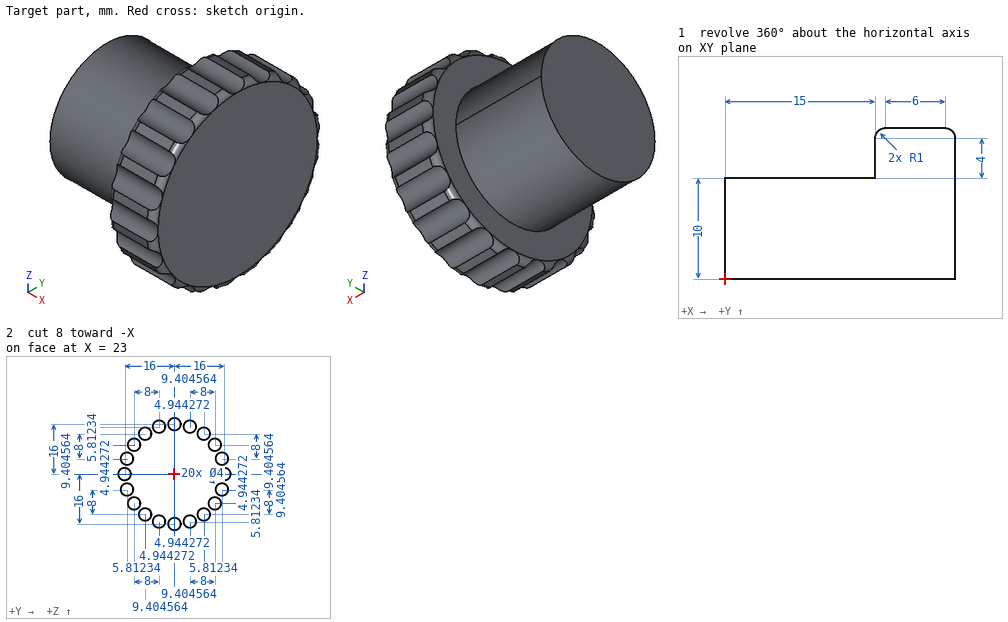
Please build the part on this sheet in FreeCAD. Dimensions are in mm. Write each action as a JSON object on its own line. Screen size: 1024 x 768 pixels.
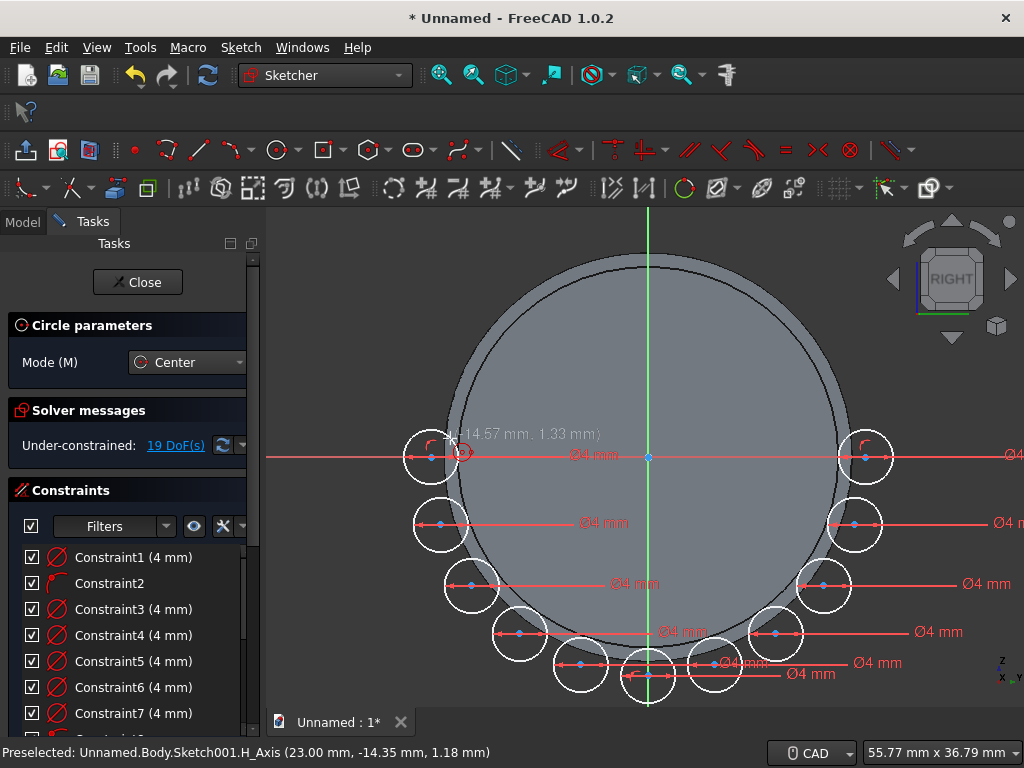
{"action": "left_click", "coordinate": [441, 390]}
{"action": "mouse_move", "coordinate": [460, 371]}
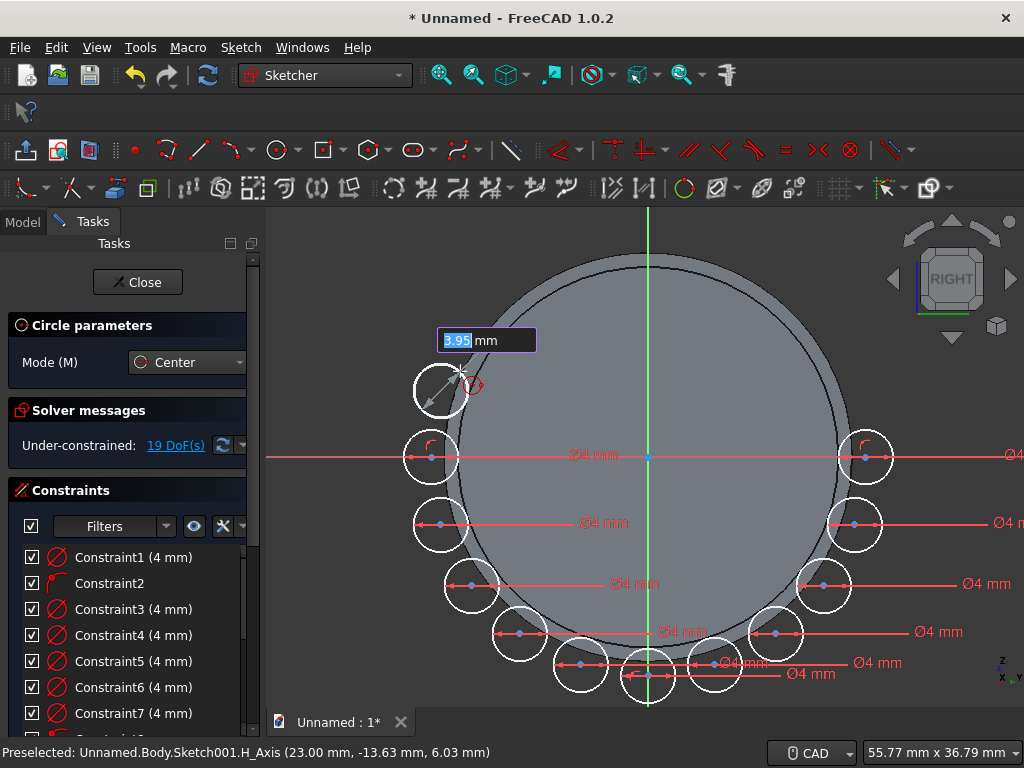
{"action": "type", "text": "4"}
{"action": "key", "text": "Return"}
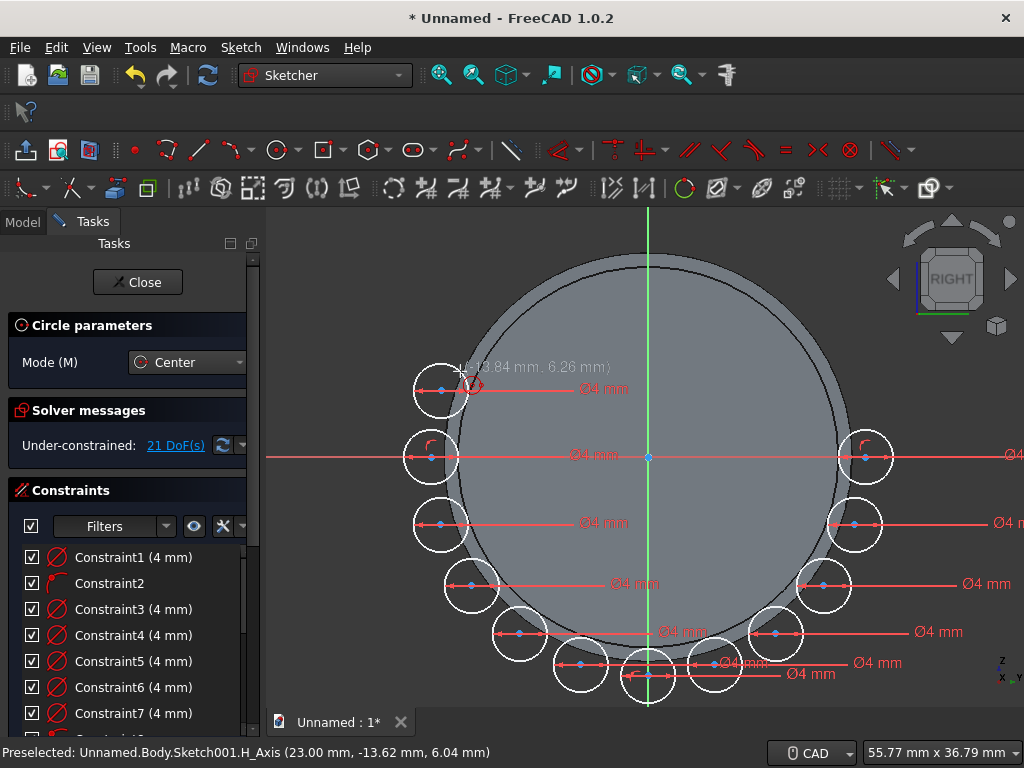
{"action": "left_click", "coordinate": [472, 329]}
{"action": "mouse_move", "coordinate": [491, 310]}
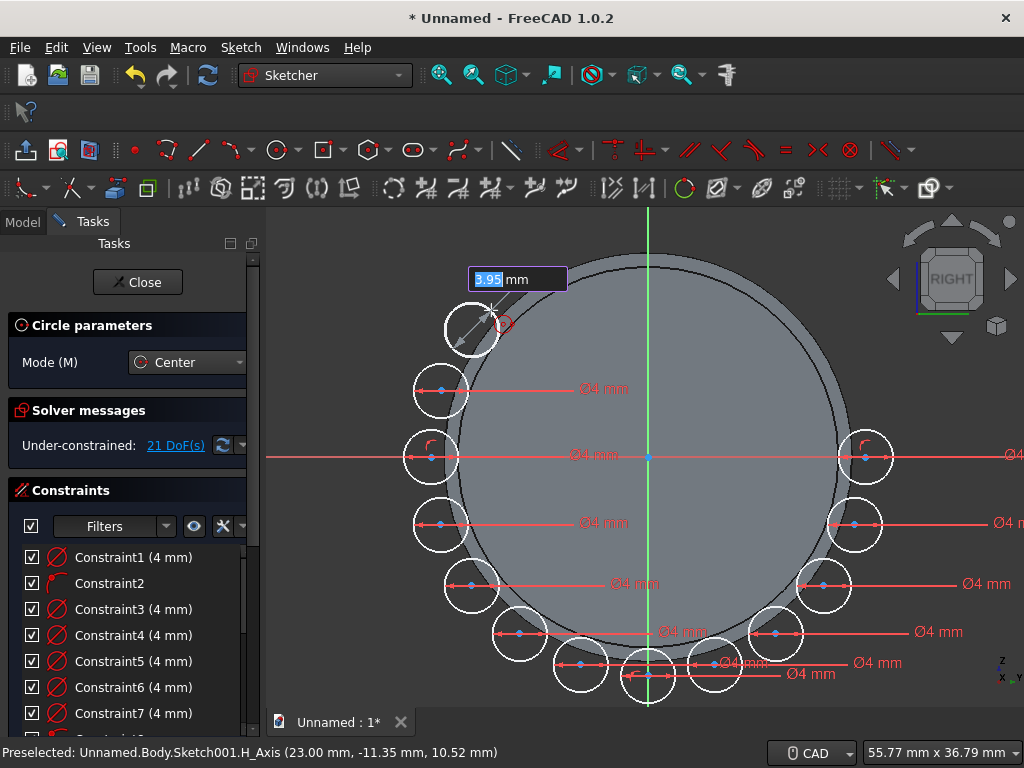
{"action": "type", "text": "4"}
{"action": "key", "text": "Return"}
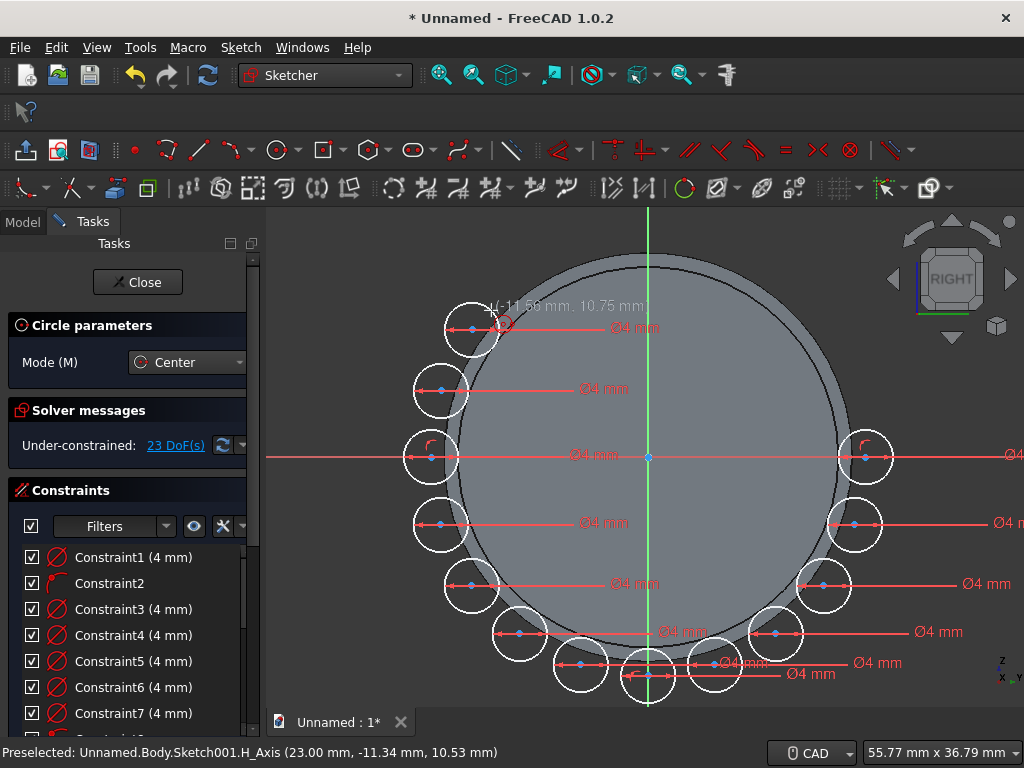
{"action": "left_click", "coordinate": [520, 281]}
{"action": "mouse_move", "coordinate": [539, 262]}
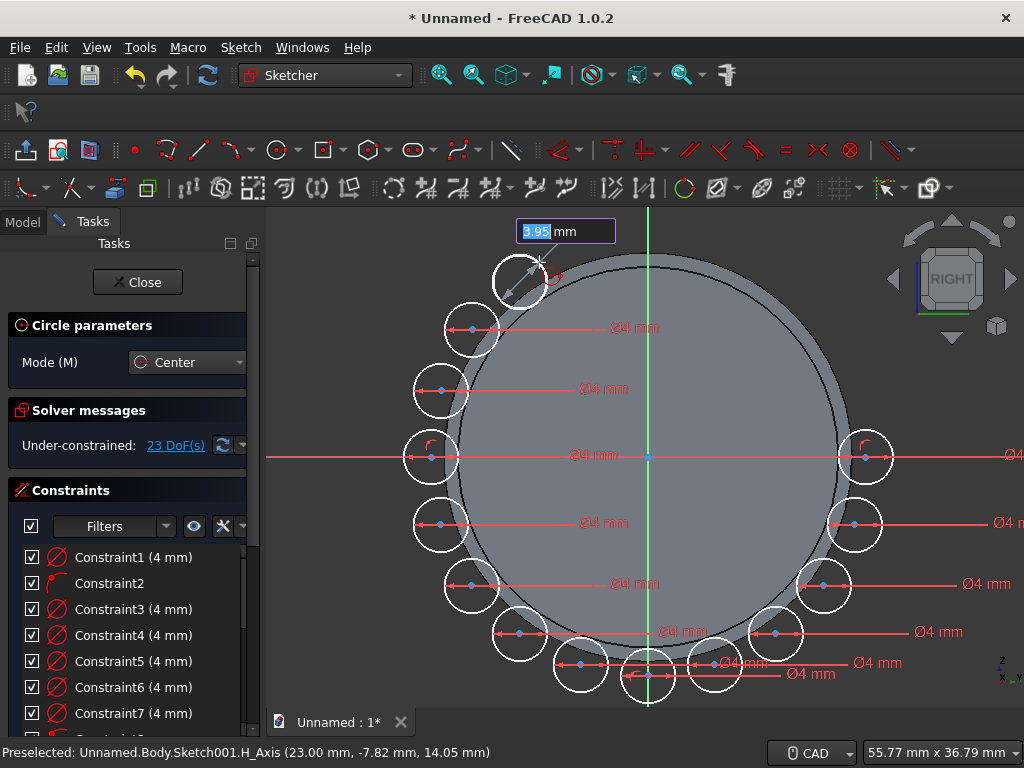
{"action": "type", "text": "4"}
{"action": "key", "text": "Return"}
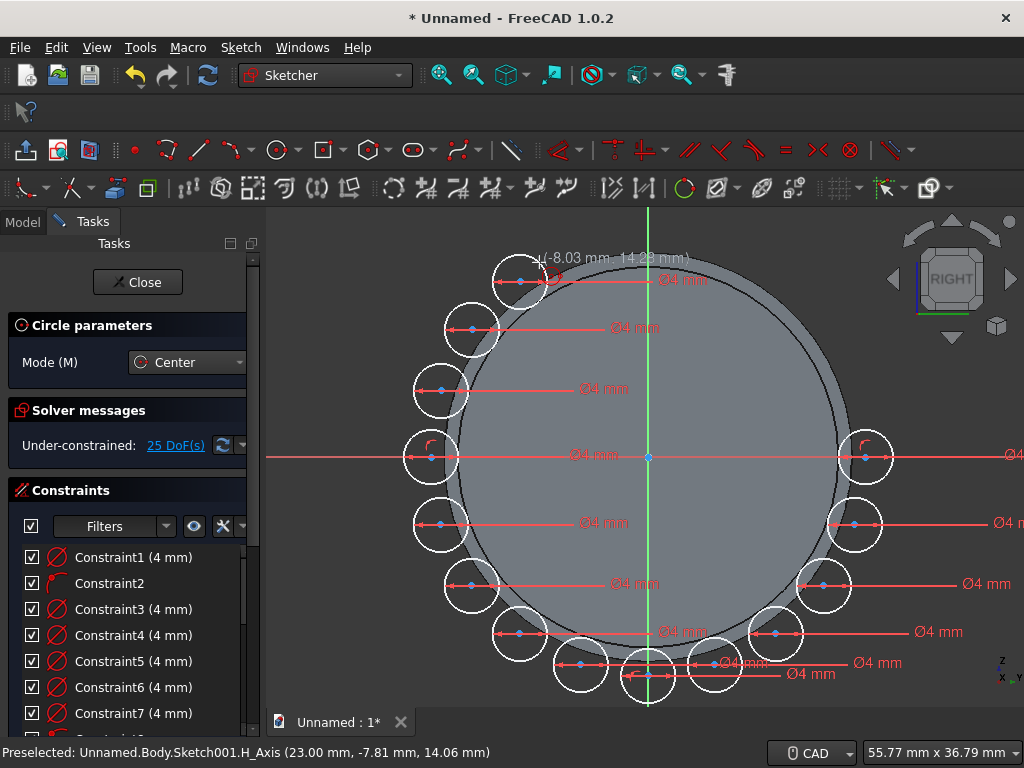
{"action": "left_click", "coordinate": [581, 250]}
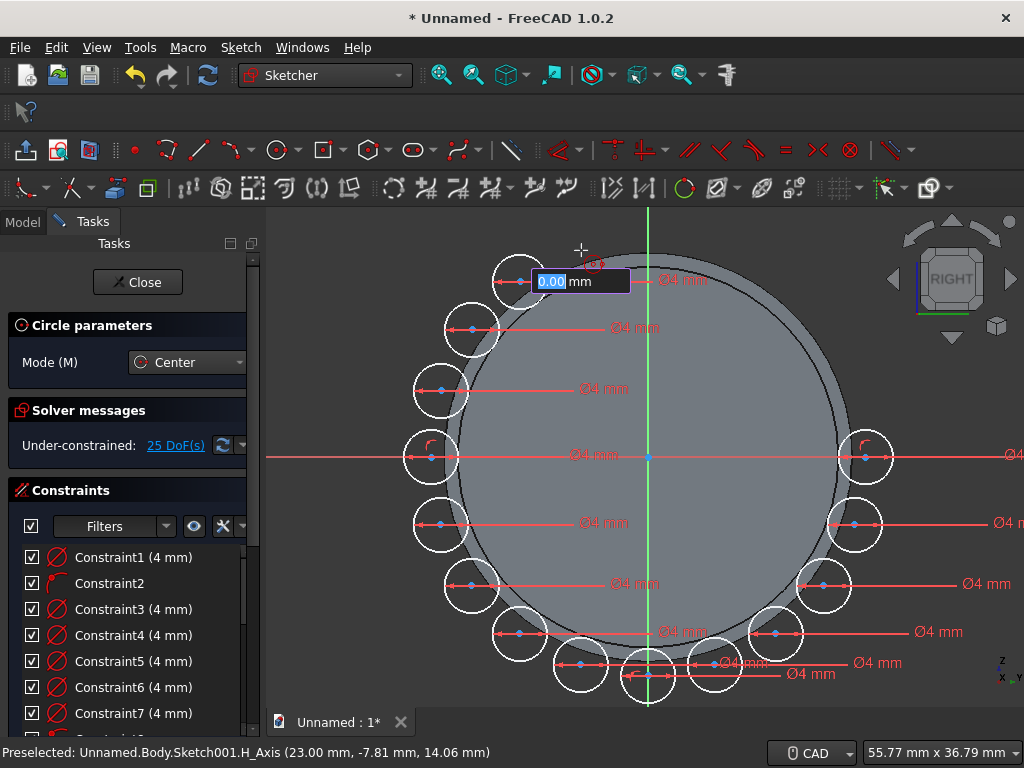
{"action": "scroll", "coordinate": [431, 457], "scroll_direction": "down", "scroll_amount": 2}
{"action": "mouse_move", "coordinate": [544, 306]}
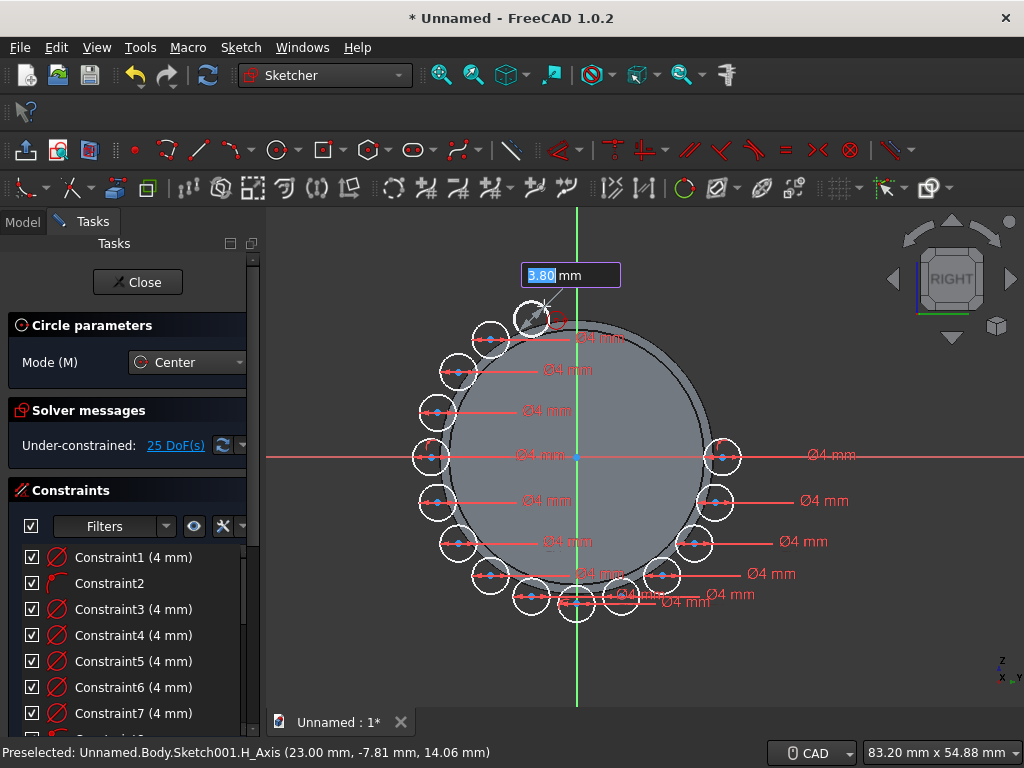
{"action": "type", "text": "4"}
{"action": "key", "text": "Return"}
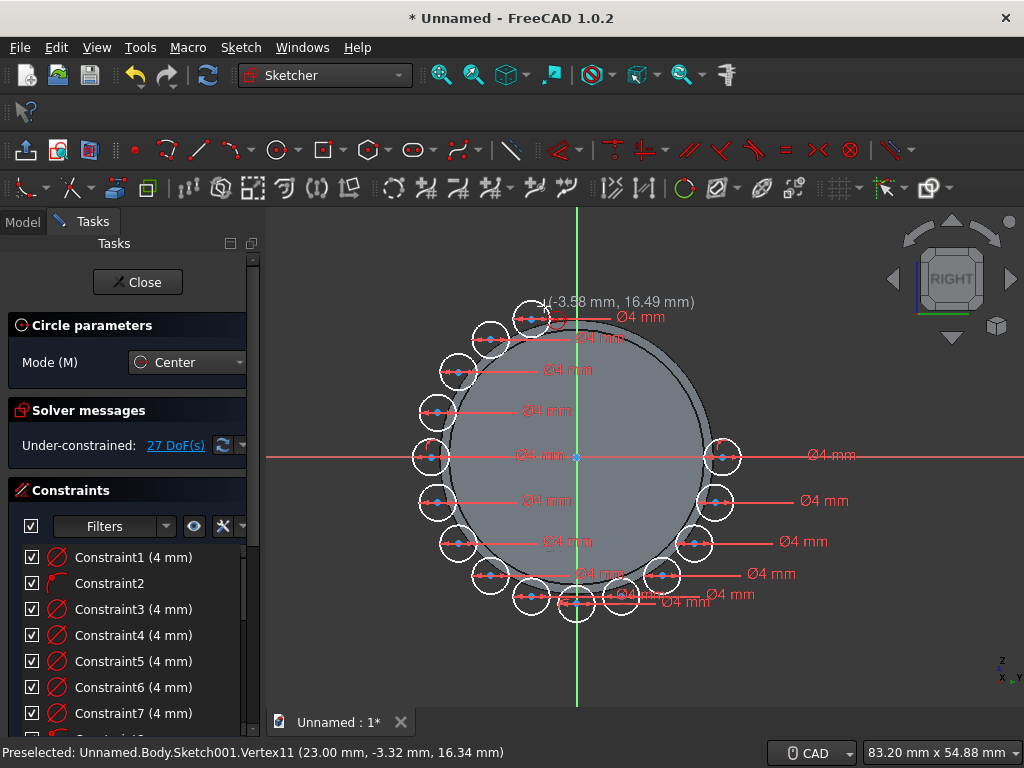
{"action": "scroll", "coordinate": [577, 311], "scroll_direction": "up", "scroll_amount": 2}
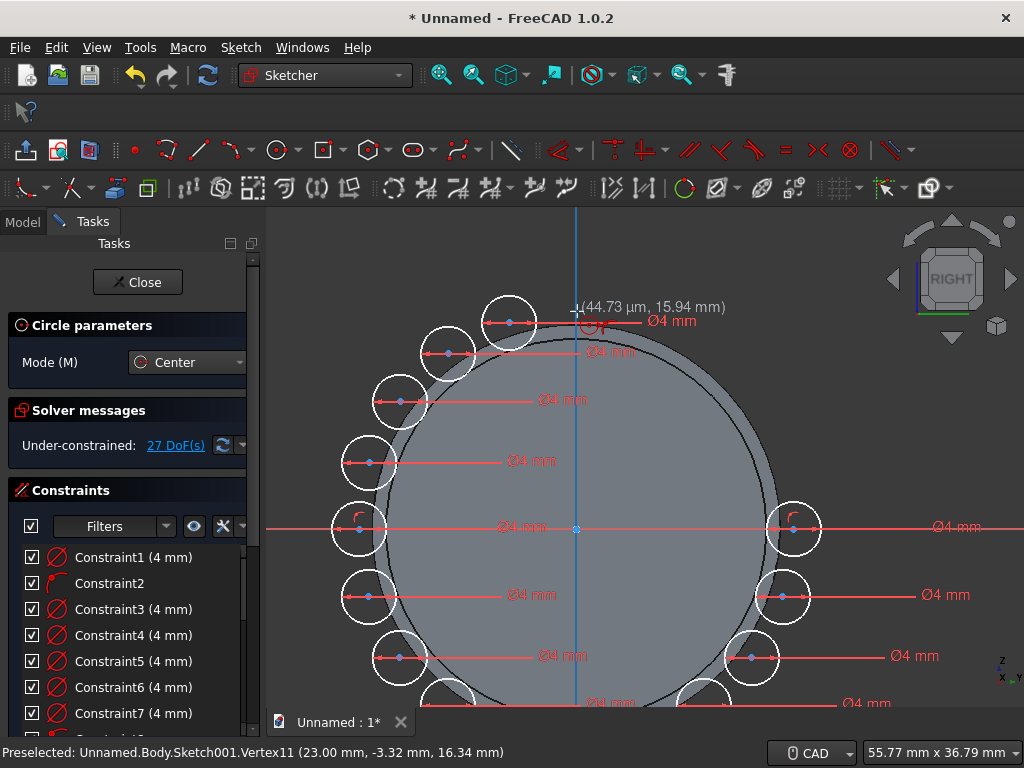
{"action": "left_click", "coordinate": [576, 312]}
{"action": "mouse_move", "coordinate": [595, 292]}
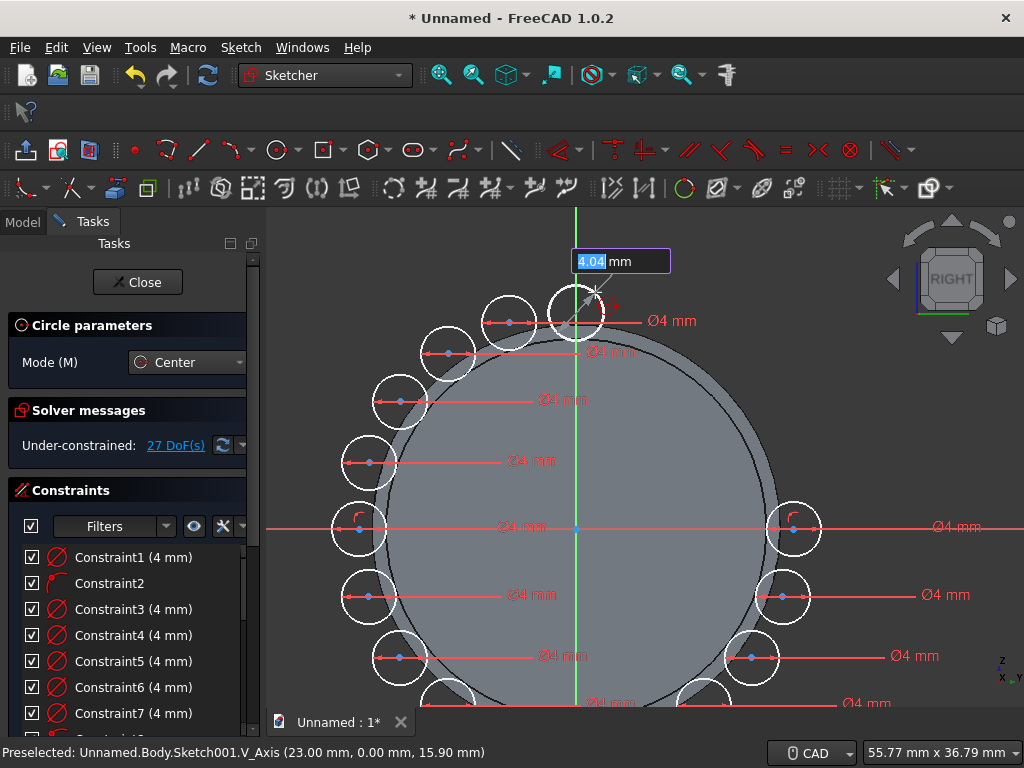
{"action": "type", "text": "4"}
{"action": "key", "text": "Return"}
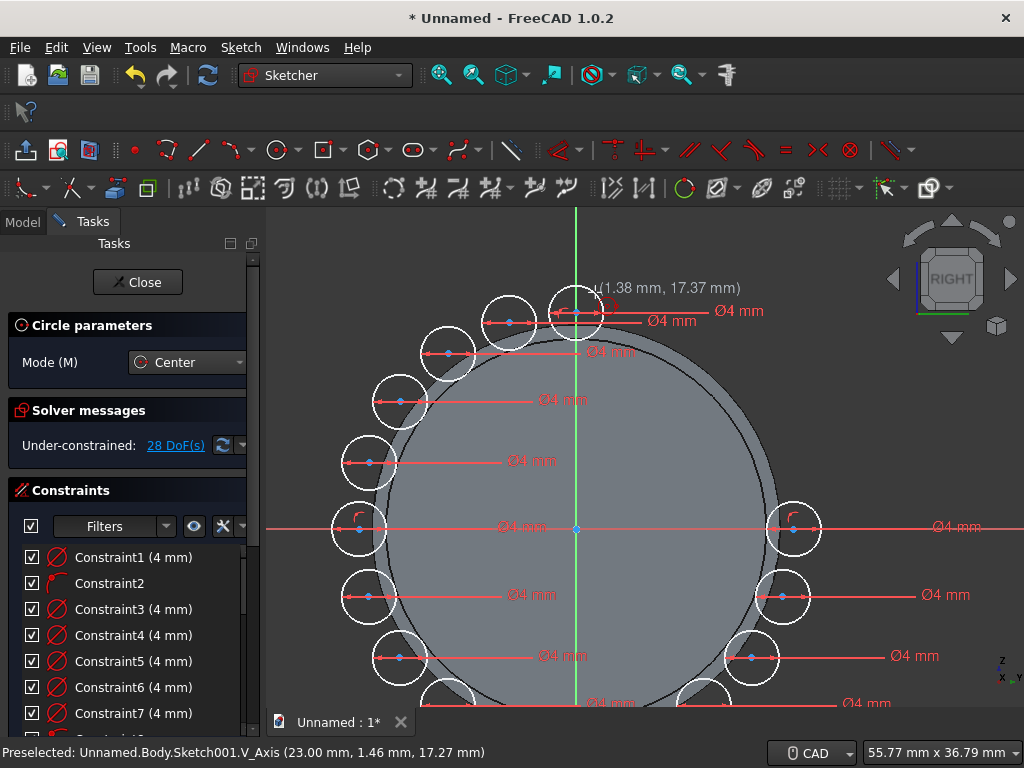
{"action": "left_click", "coordinate": [643, 322]}
{"action": "mouse_move", "coordinate": [663, 303]}